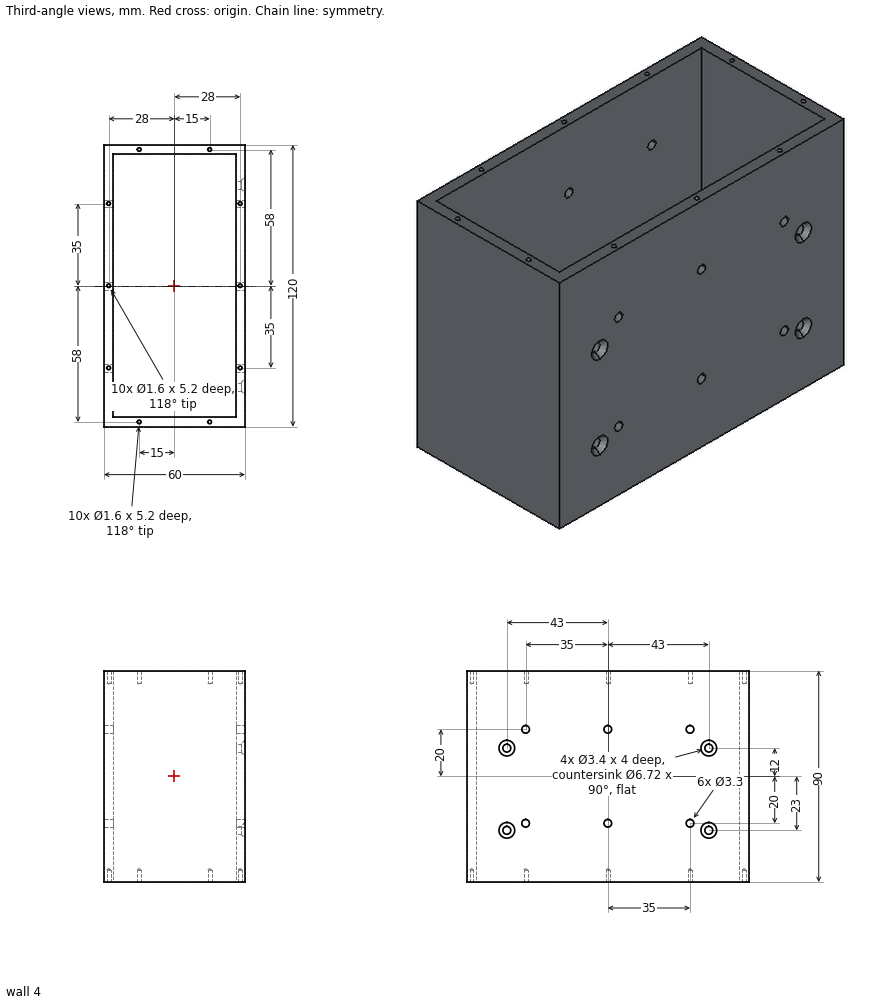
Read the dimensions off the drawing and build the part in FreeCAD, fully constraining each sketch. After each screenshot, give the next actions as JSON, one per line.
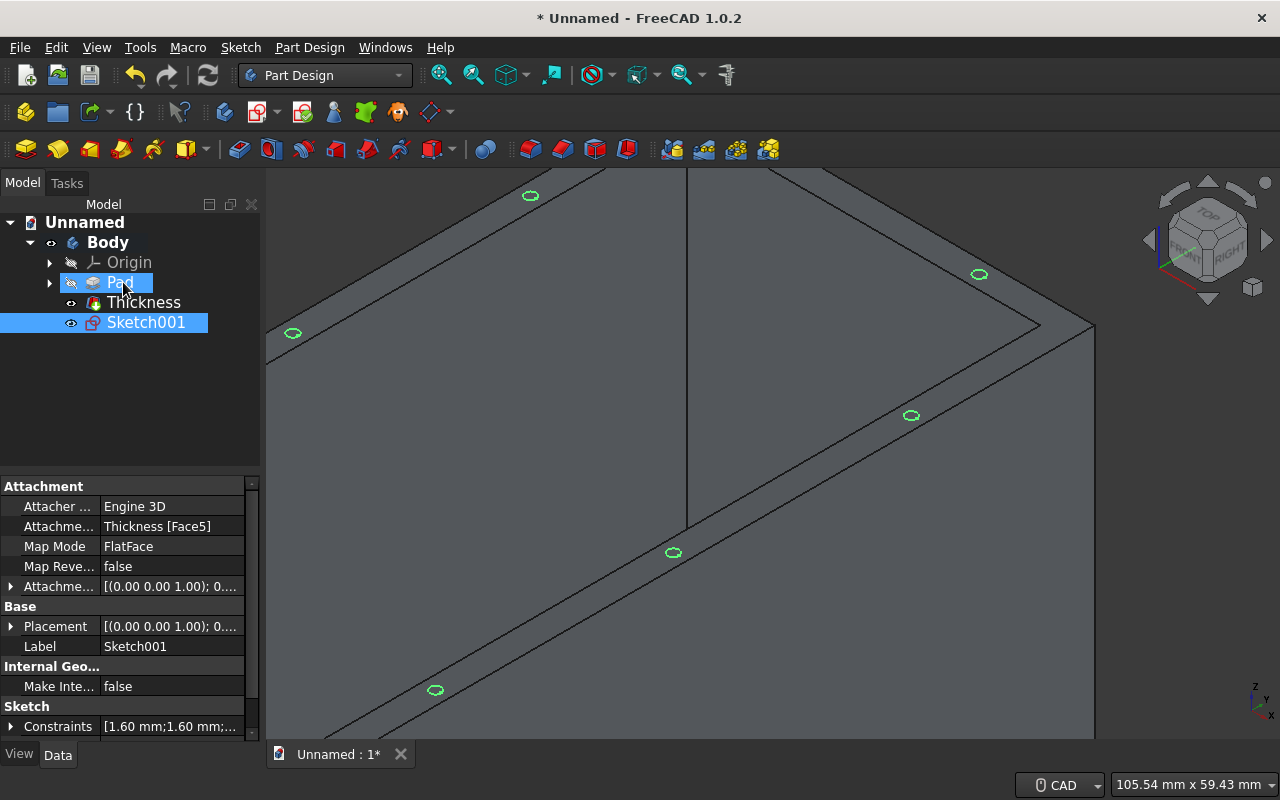
{"action": "left_click", "coordinate": [272, 150]}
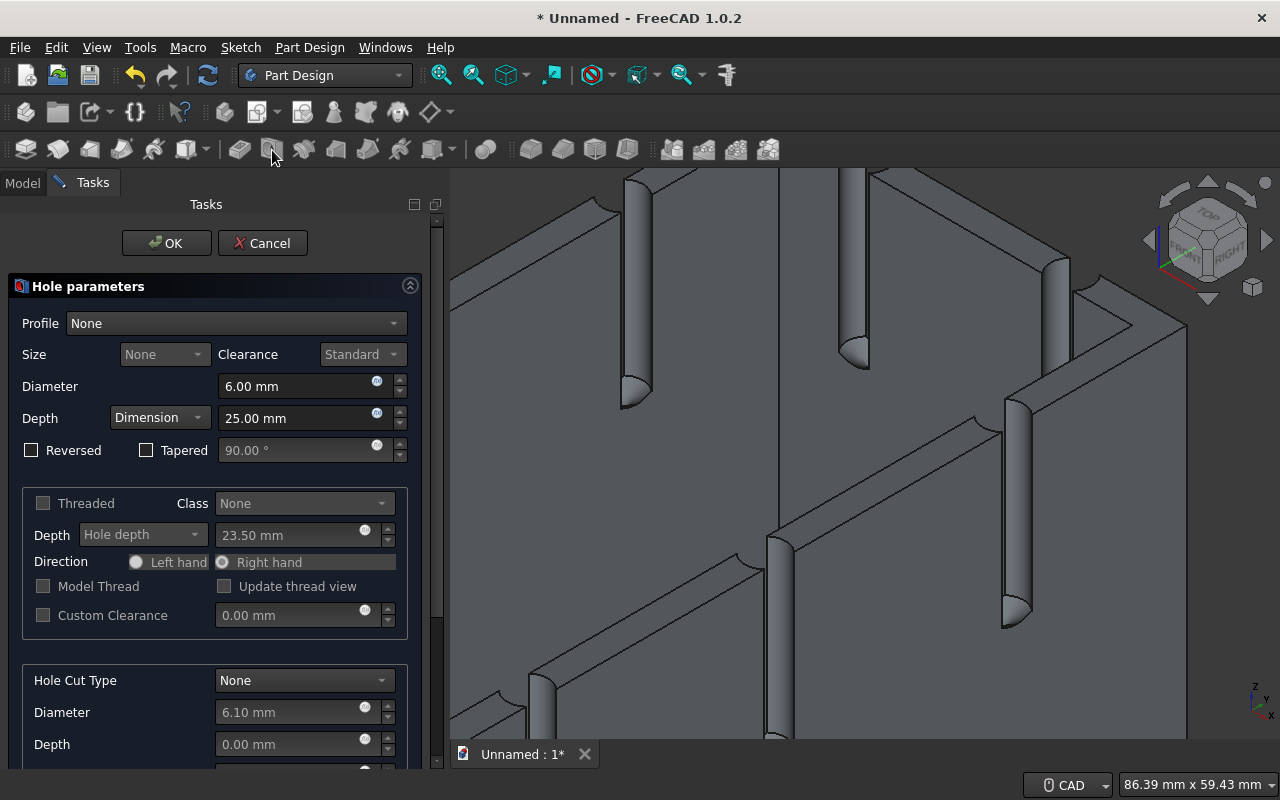
{"action": "triple_click", "coordinate": [305, 386]}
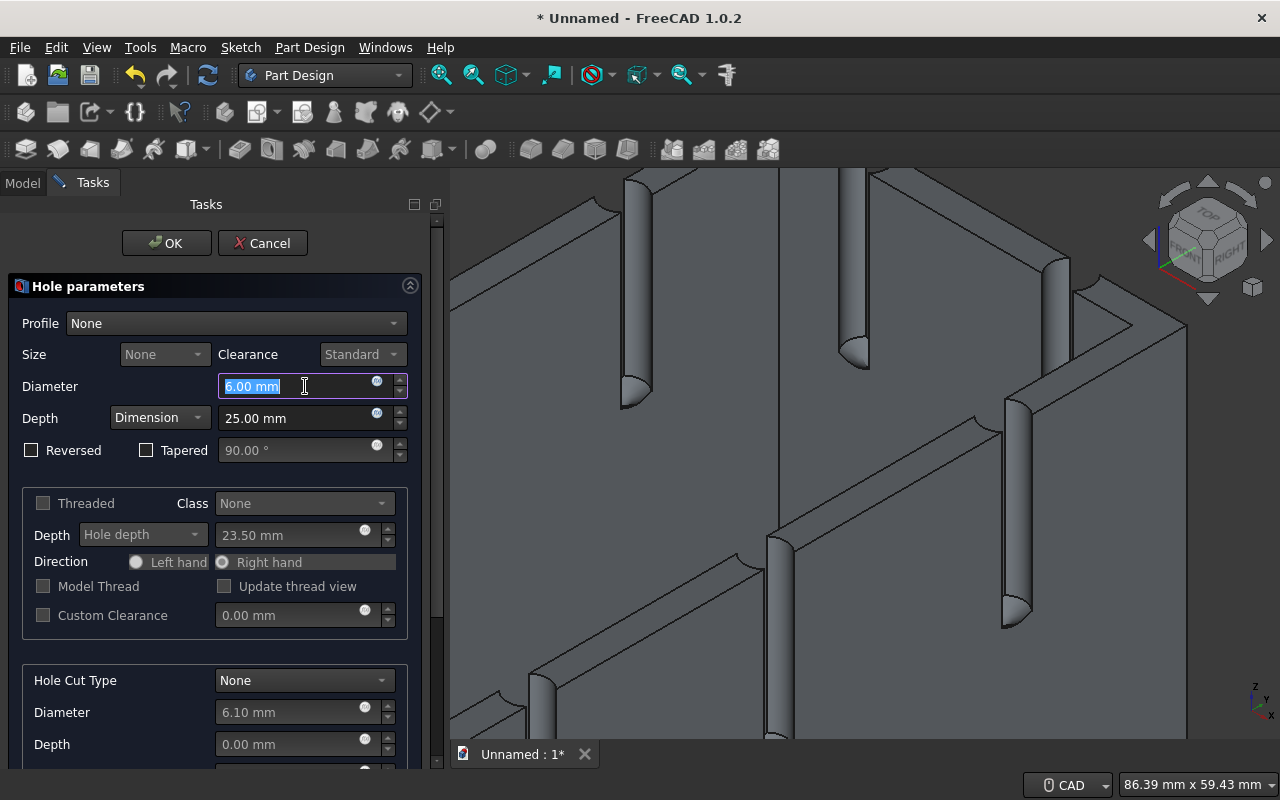
{"action": "type", "text": "1.6"}
{"action": "key", "text": "Tab"}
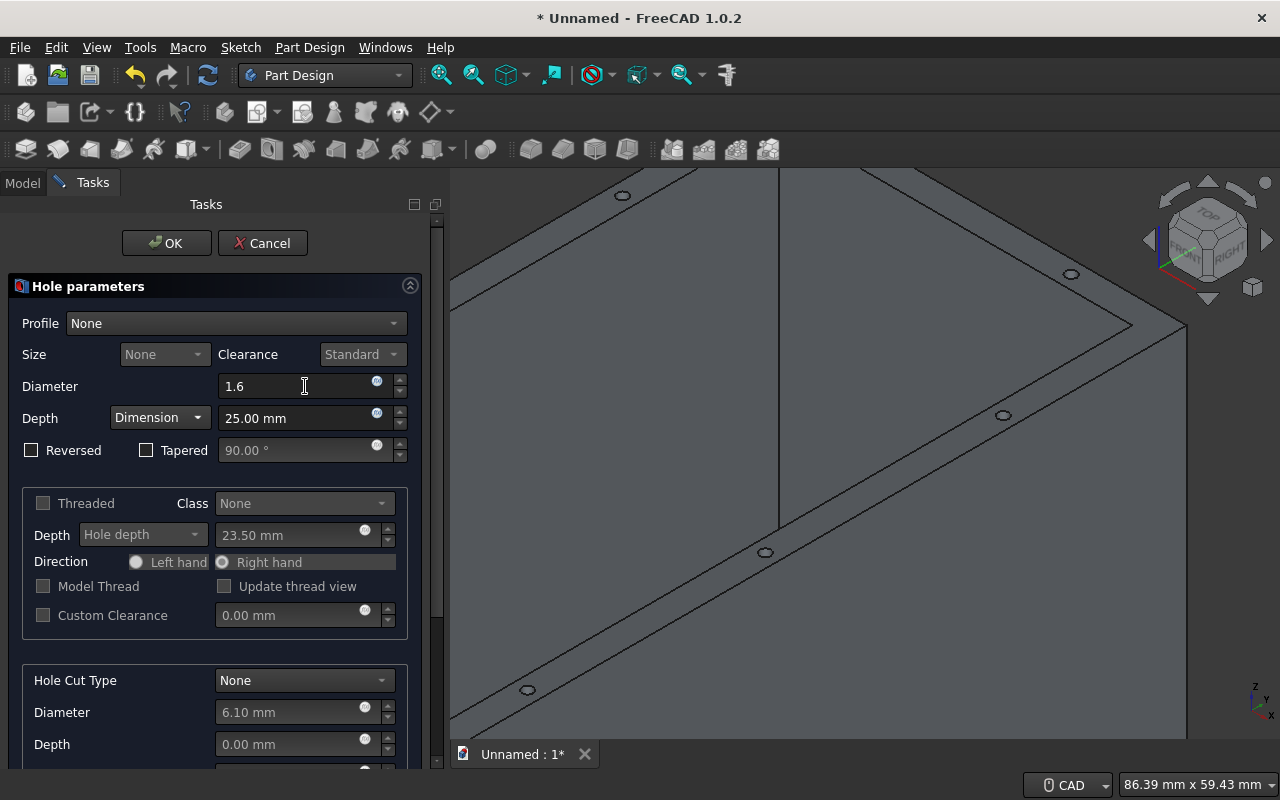
{"action": "triple_click", "coordinate": [305, 418]}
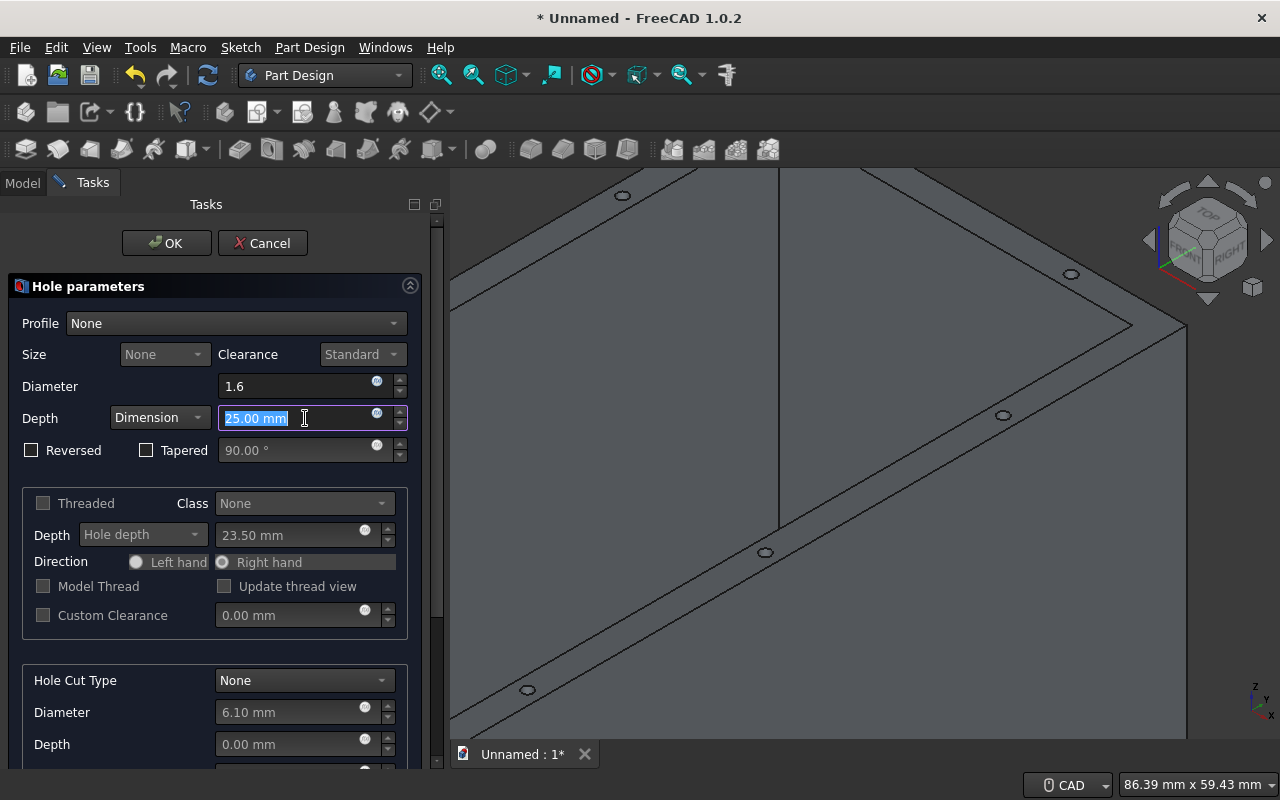
{"action": "type", "text": "5.2"}
{"action": "key", "text": "Tab"}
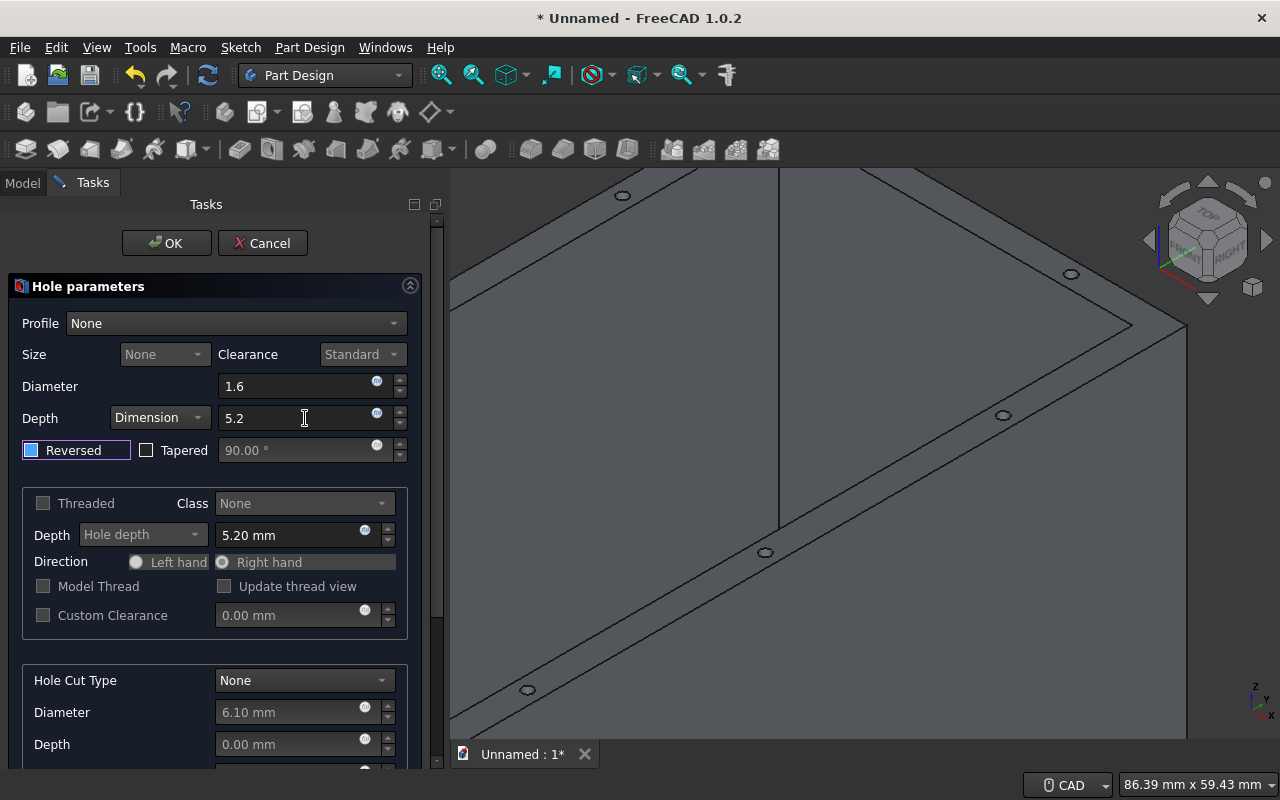
{"action": "left_click", "coordinate": [167, 243]}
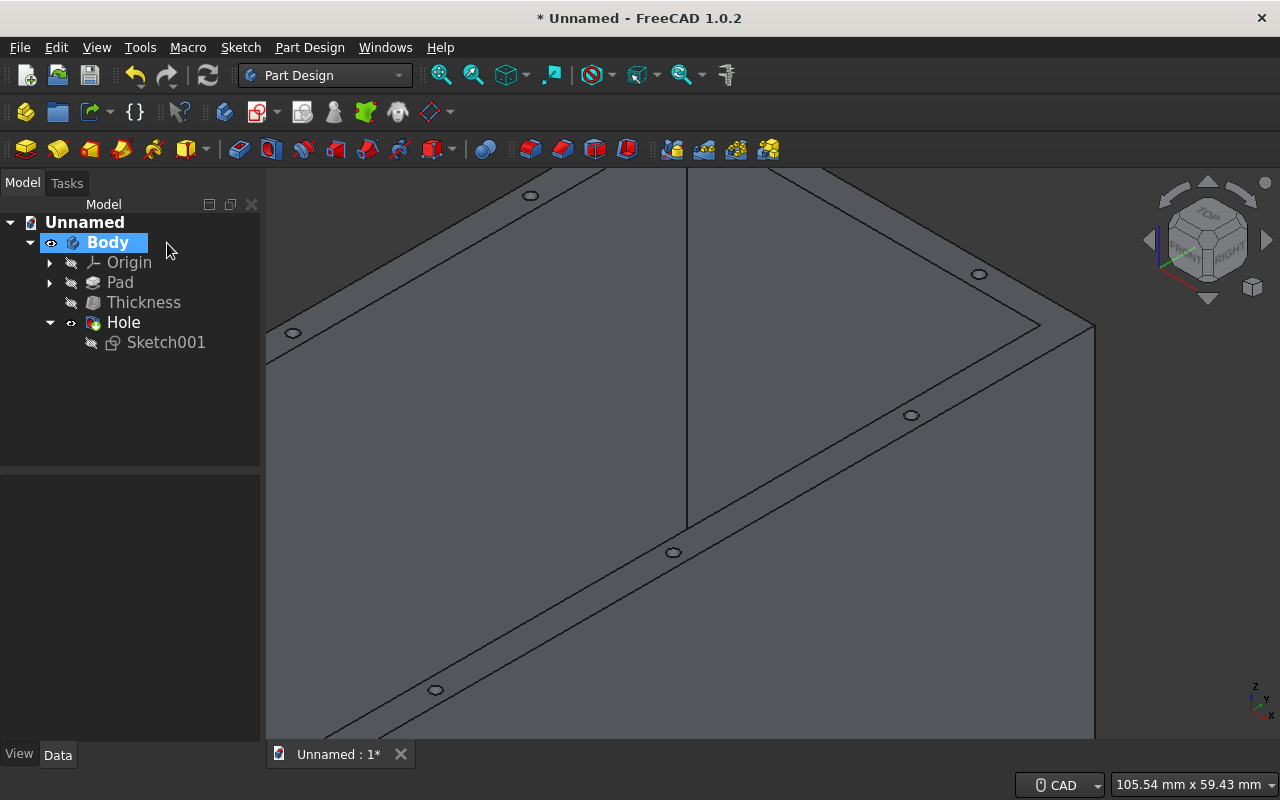
{"action": "left_click", "coordinate": [442, 76]}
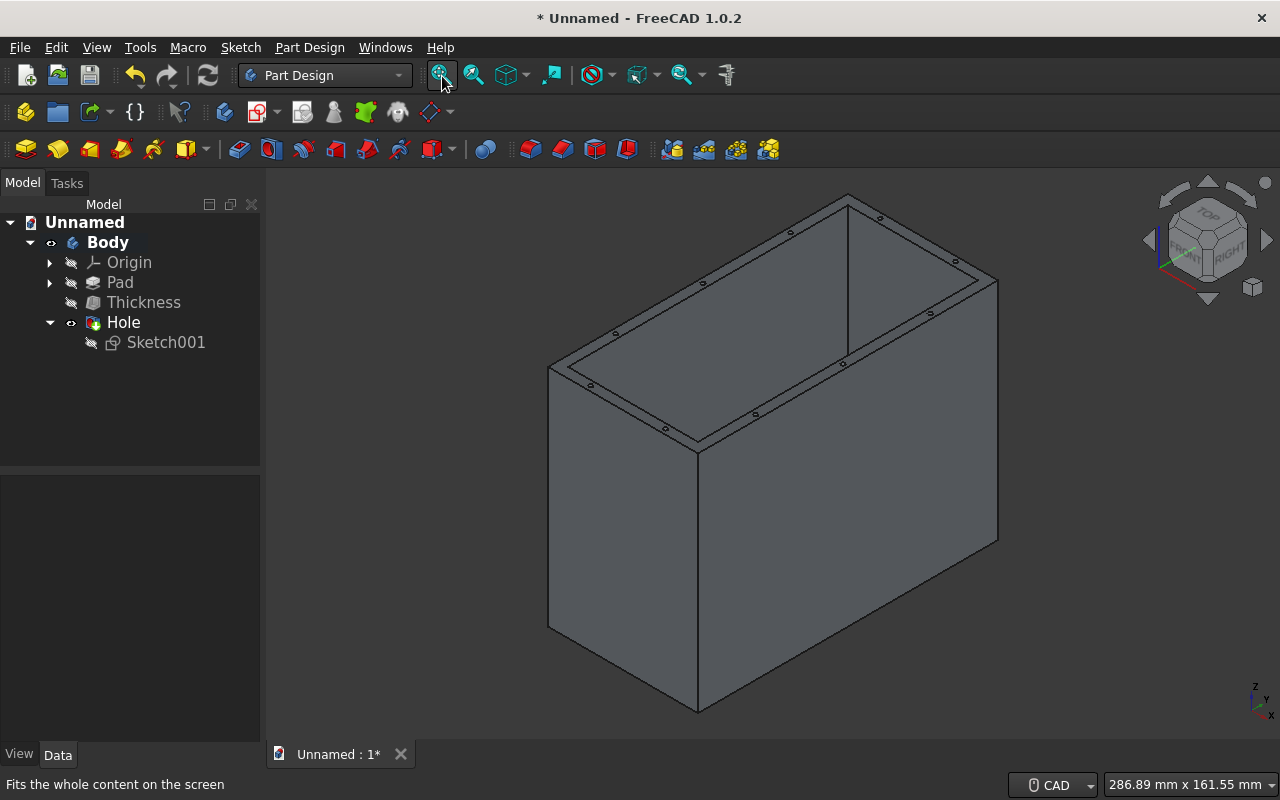
{"action": "key", "text": "5"}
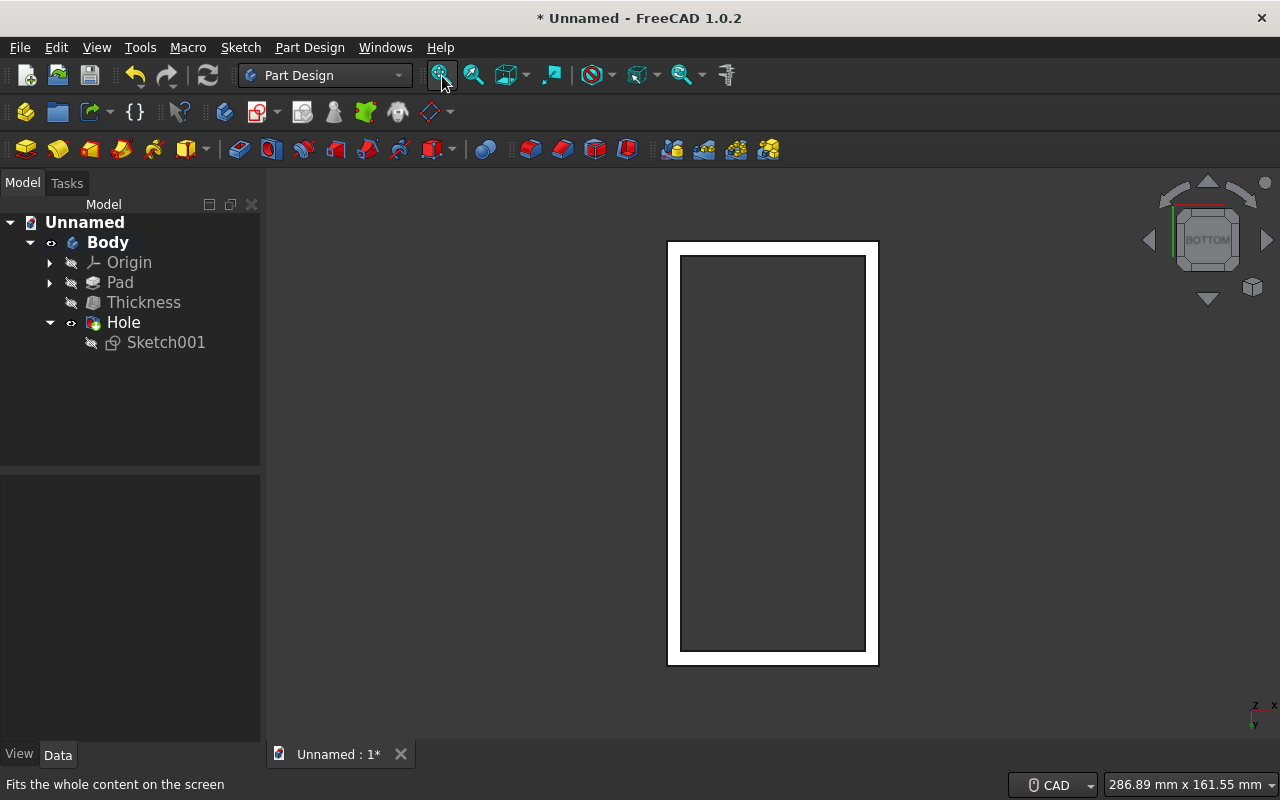
{"action": "scroll", "coordinate": [808, 655], "scroll_direction": "up", "scroll_amount": 5}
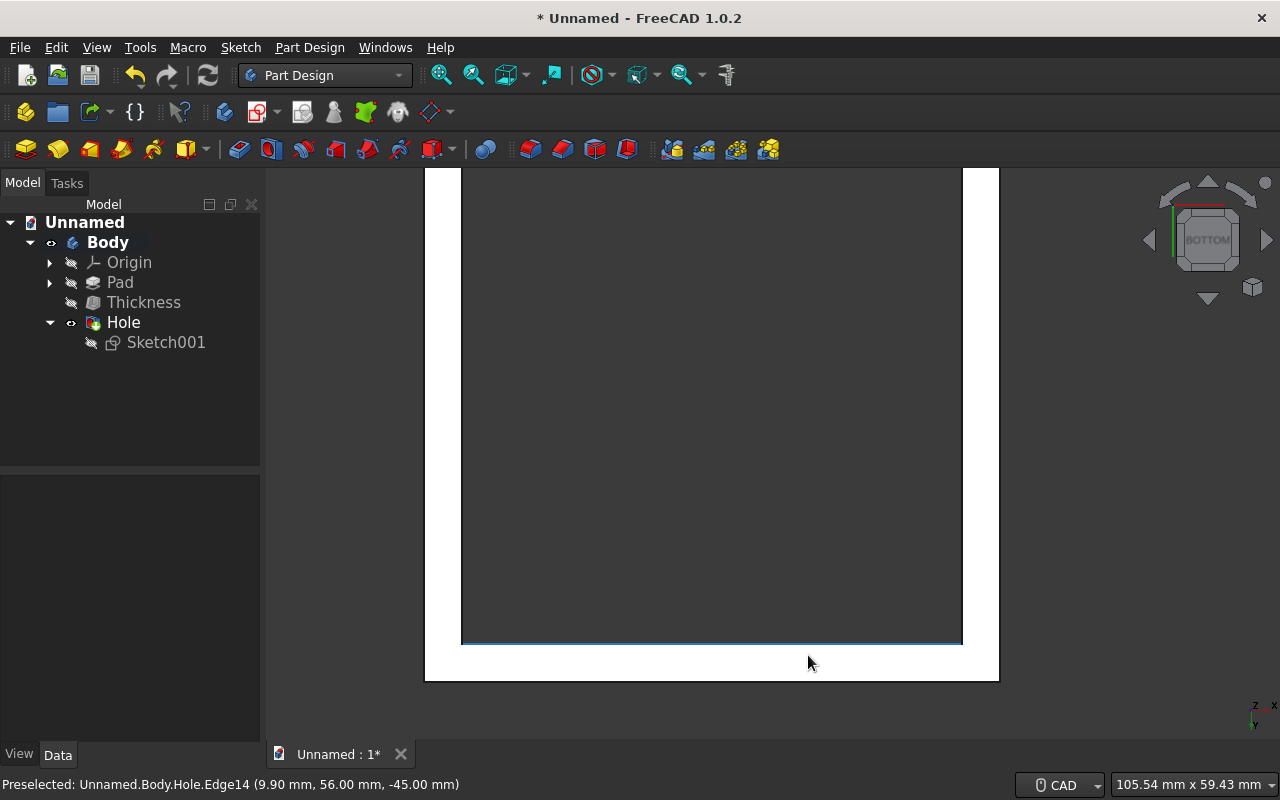
{"action": "left_click", "coordinate": [808, 656]}